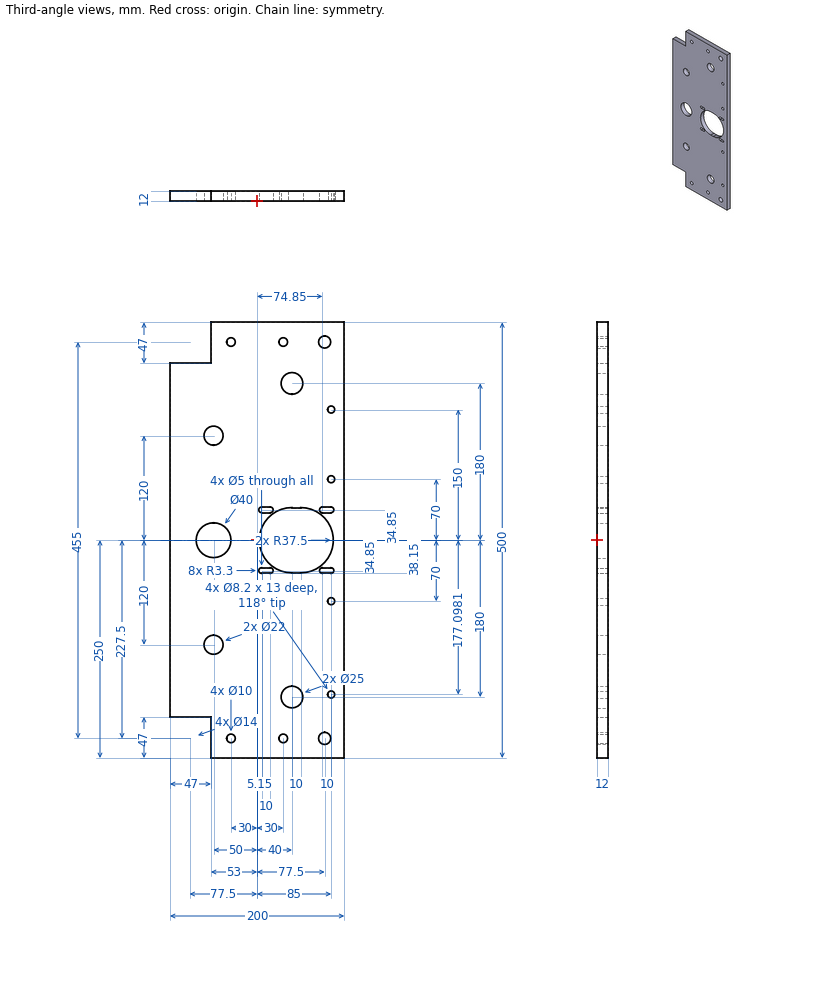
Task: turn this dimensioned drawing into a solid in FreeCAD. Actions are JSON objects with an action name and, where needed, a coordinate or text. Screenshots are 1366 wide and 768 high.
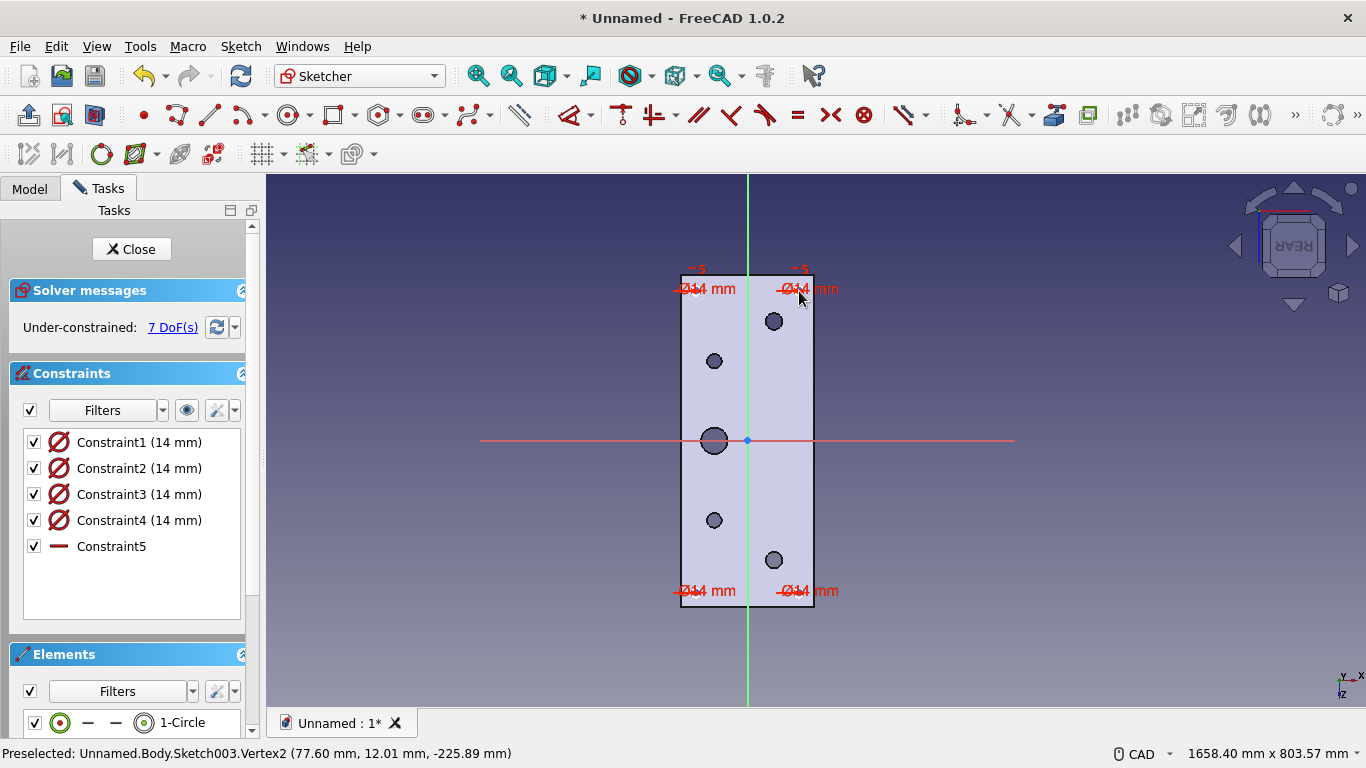
{"action": "left_click", "coordinate": [696, 291]}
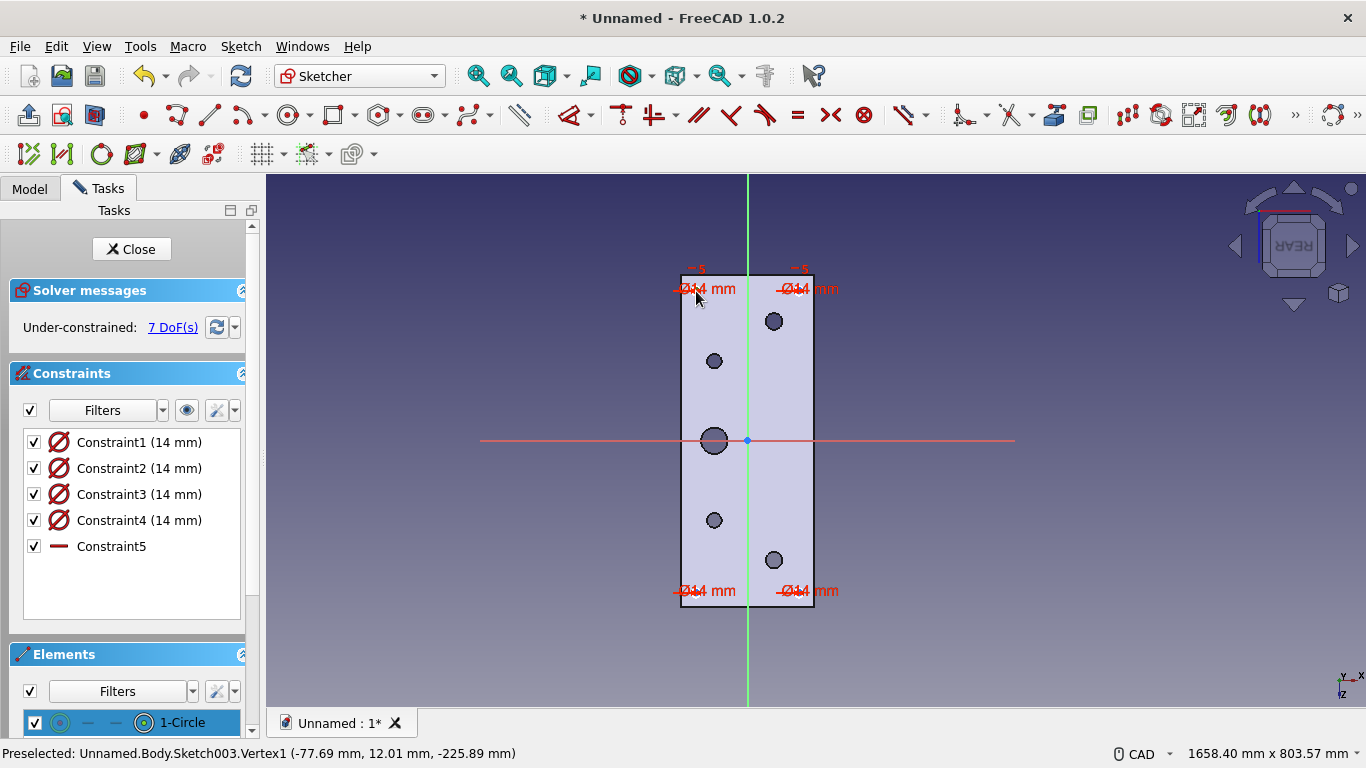
{"action": "left_click", "coordinate": [696, 593]}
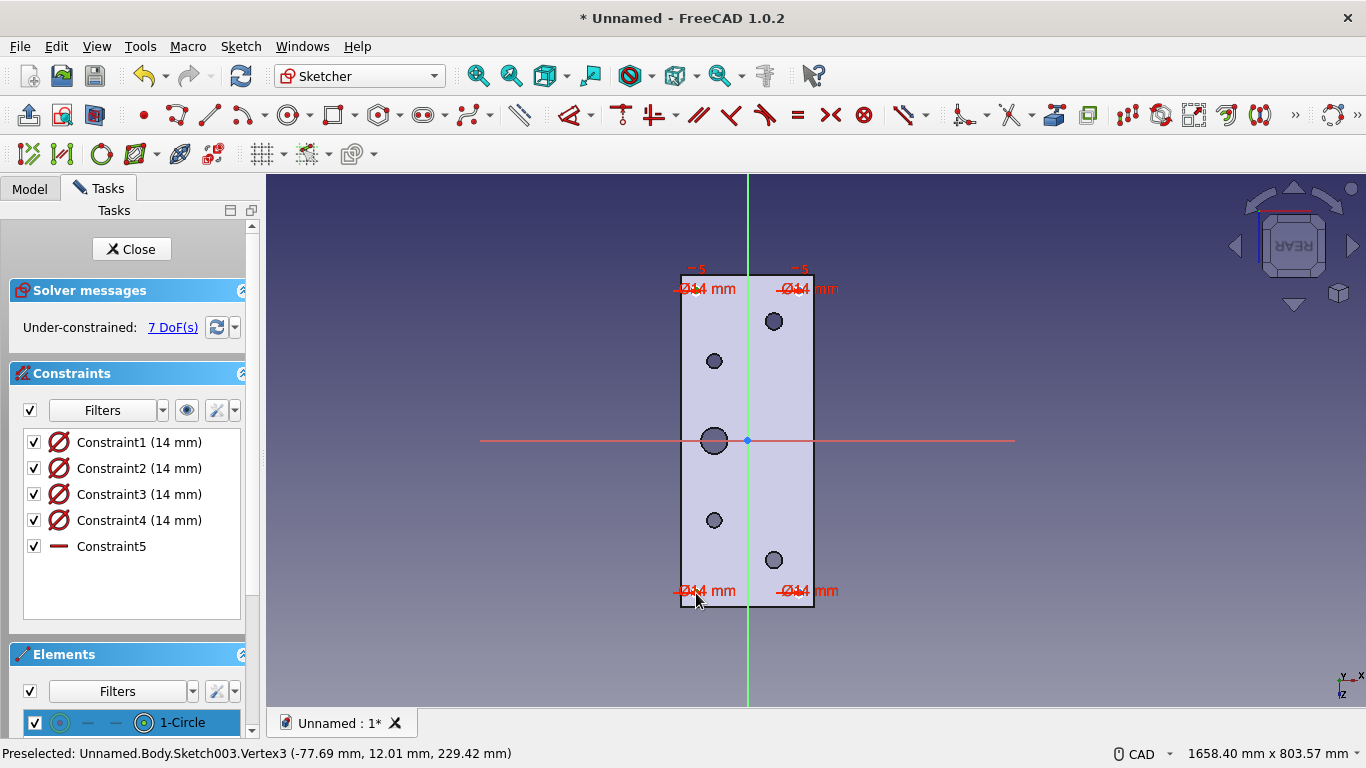
{"action": "key", "text": "v"}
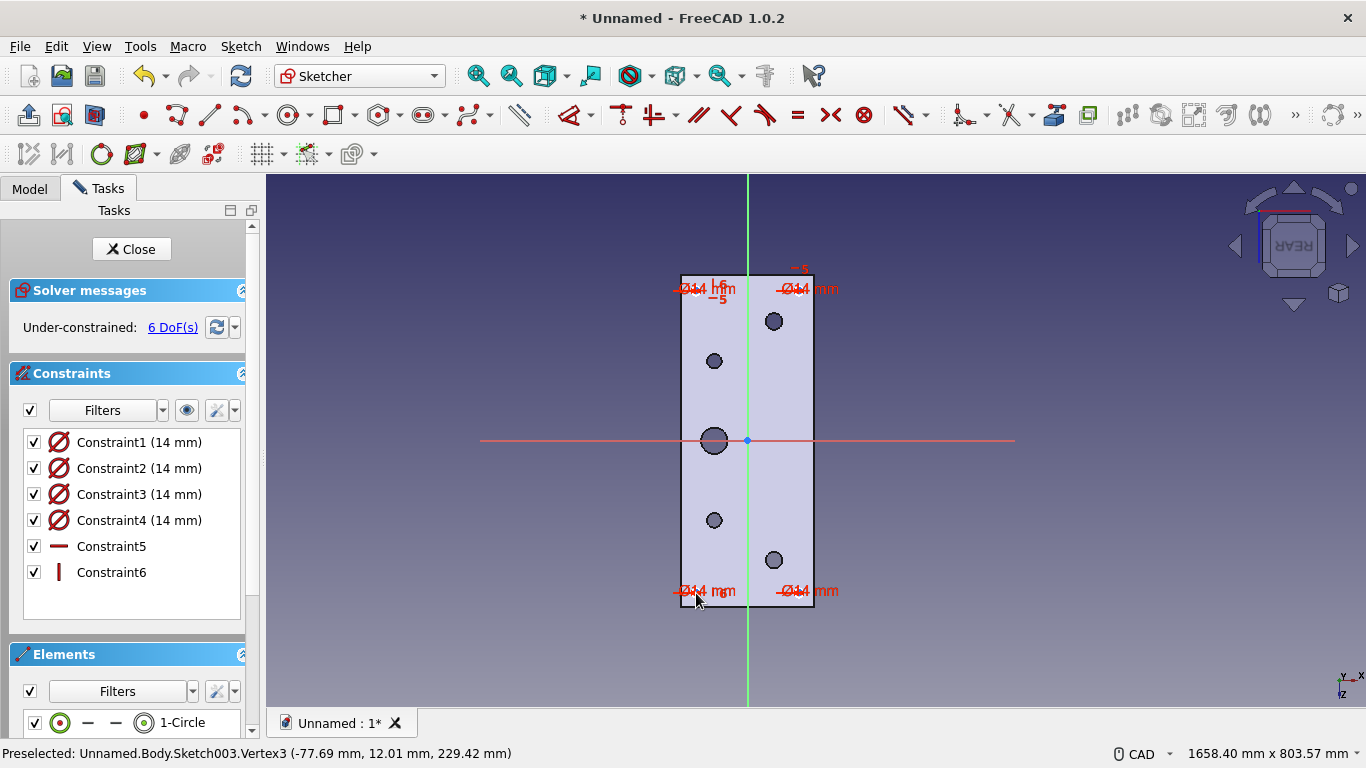
{"action": "left_click", "coordinate": [799, 291]}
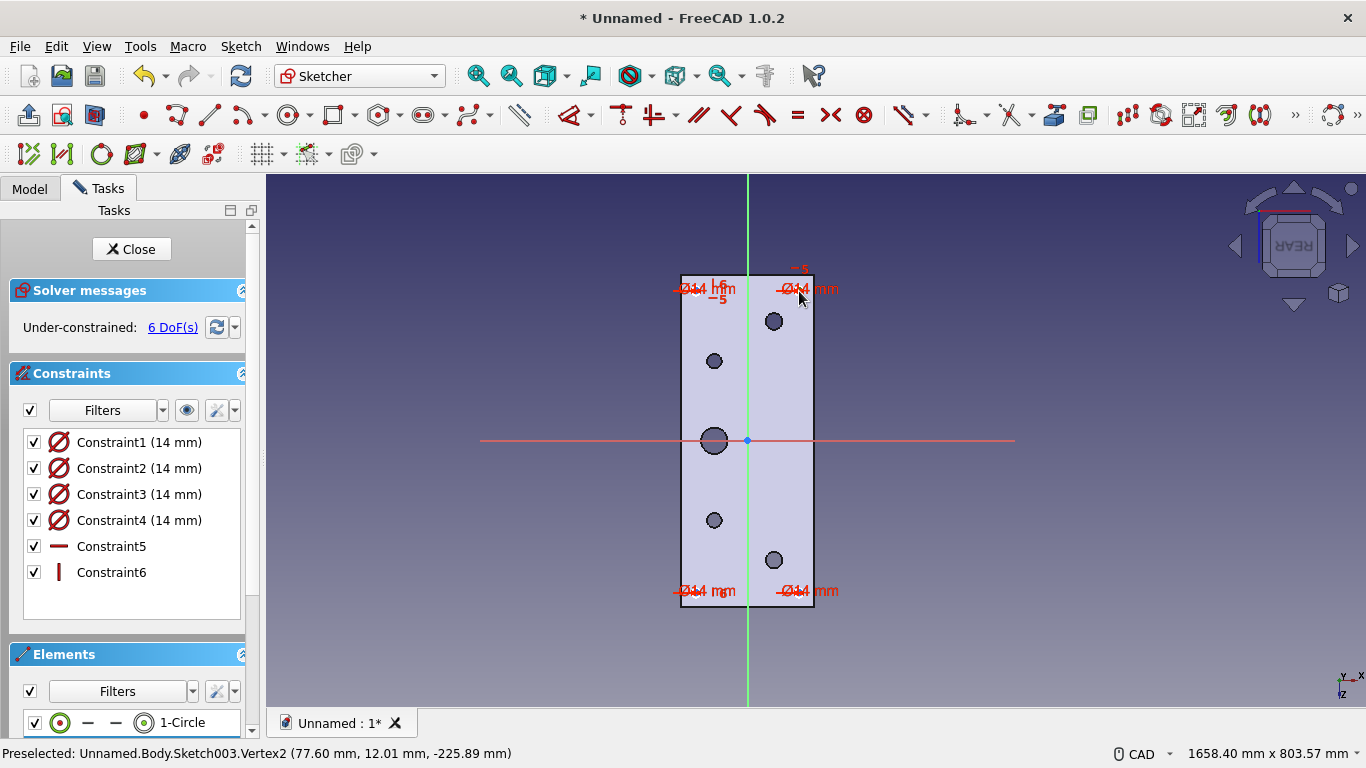
{"action": "left_click", "coordinate": [799, 593]}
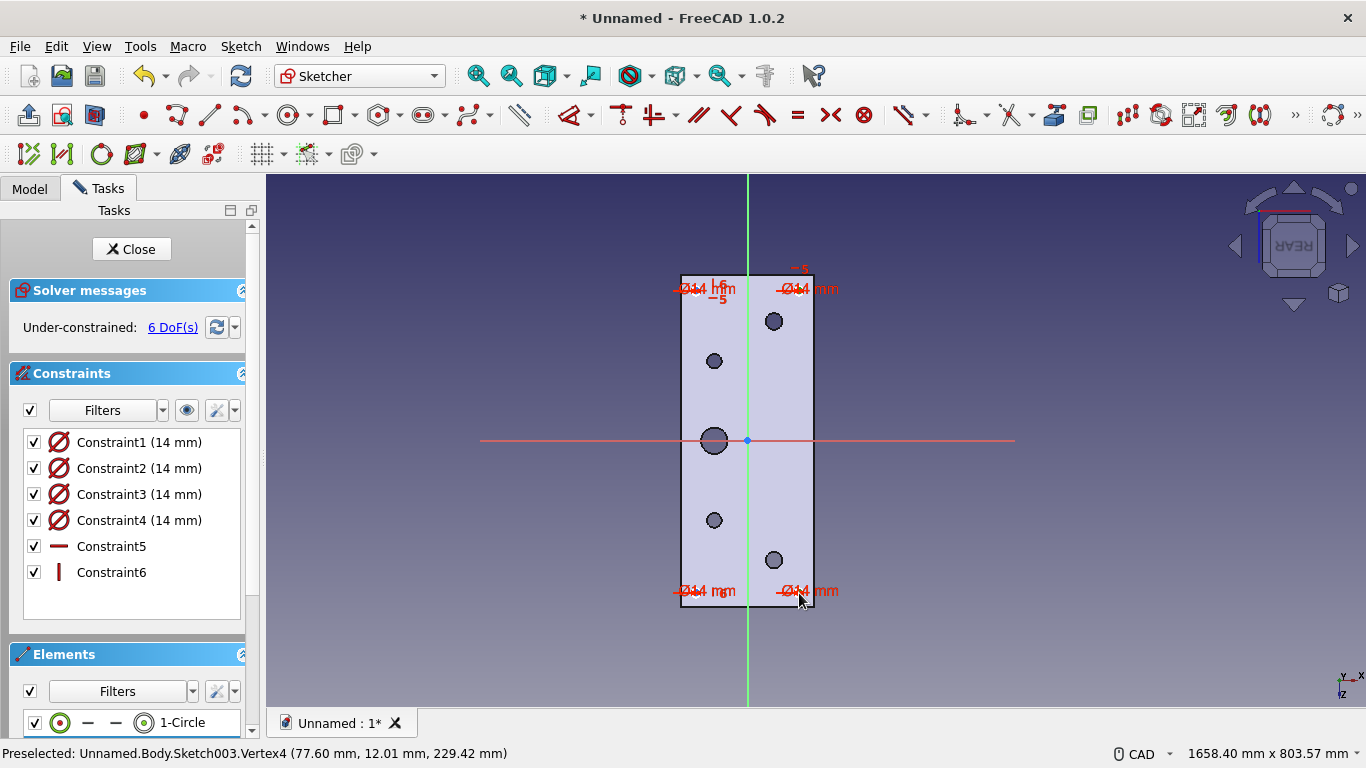
{"action": "key", "text": "v"}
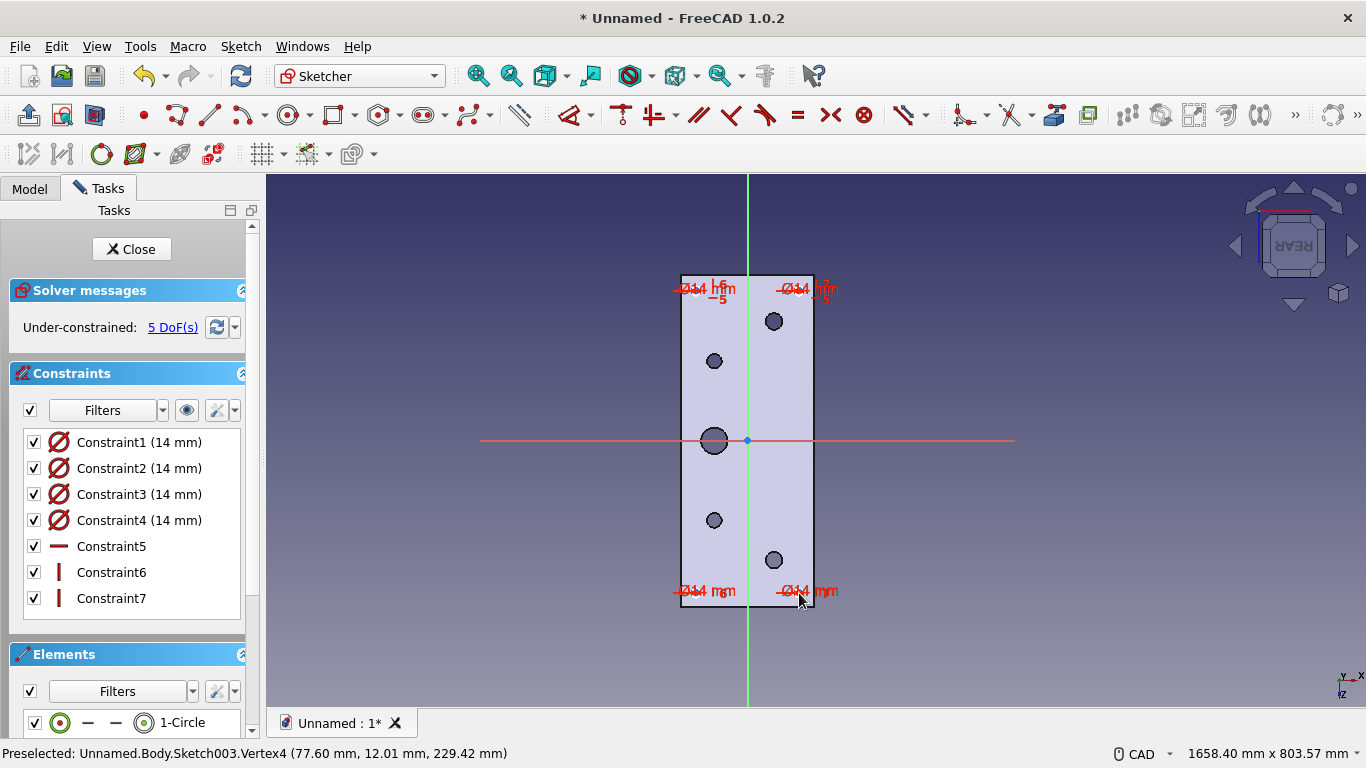
{"action": "left_click", "coordinate": [696, 593]}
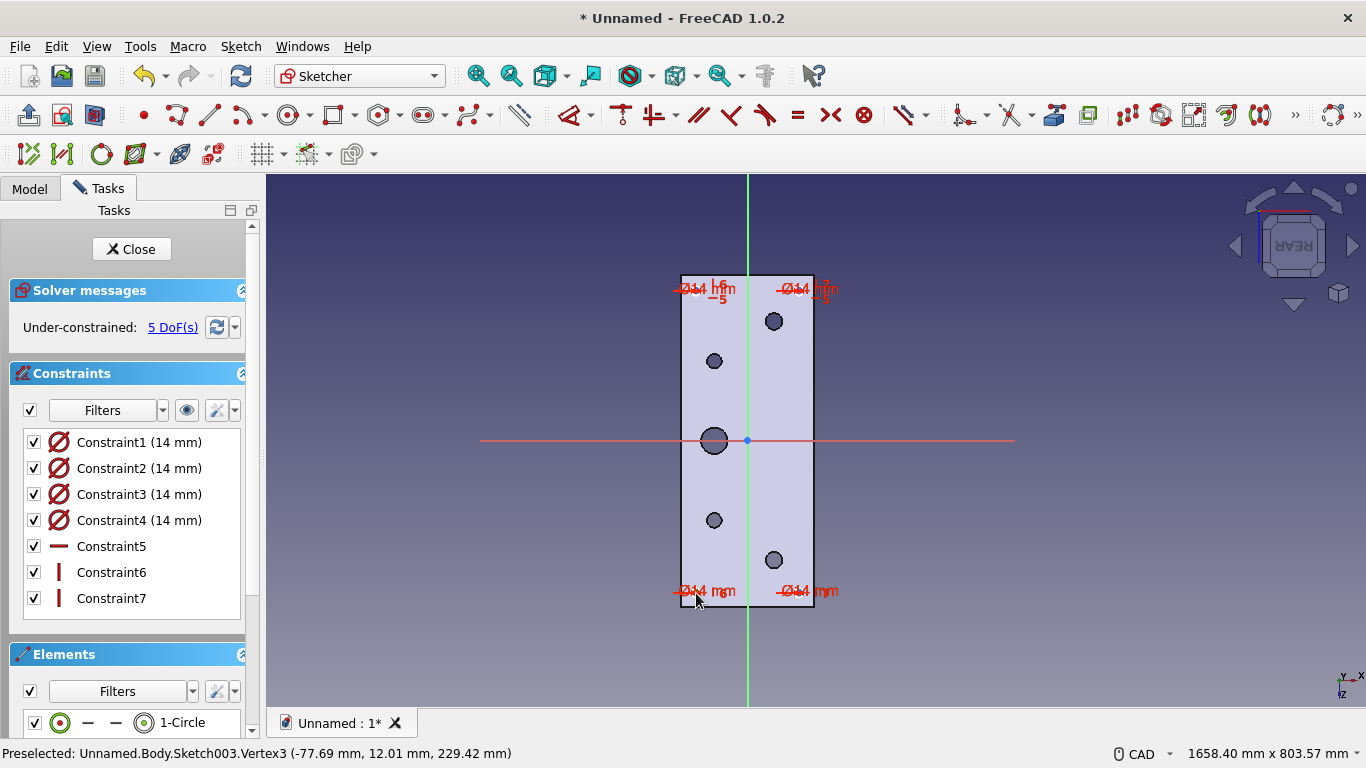
{"action": "left_click", "coordinate": [799, 593]}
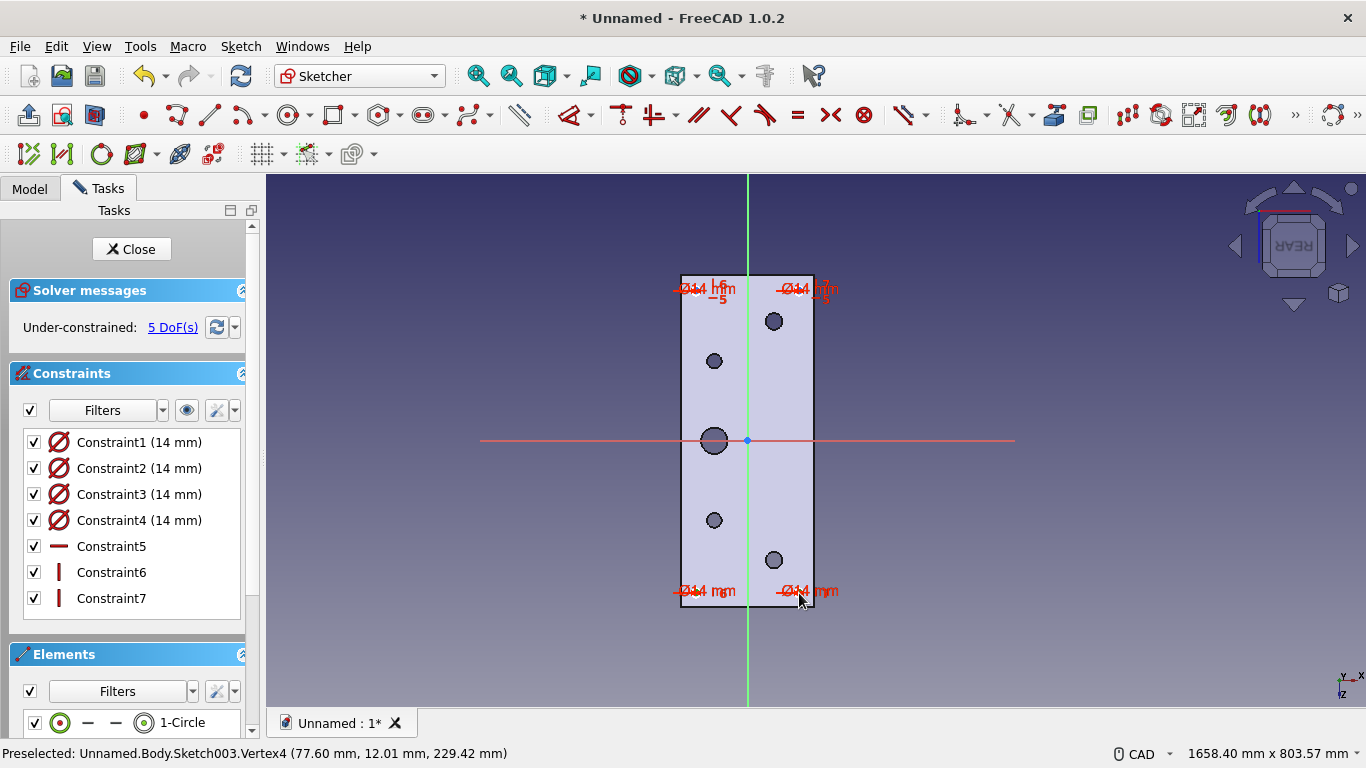
{"action": "key", "text": "h"}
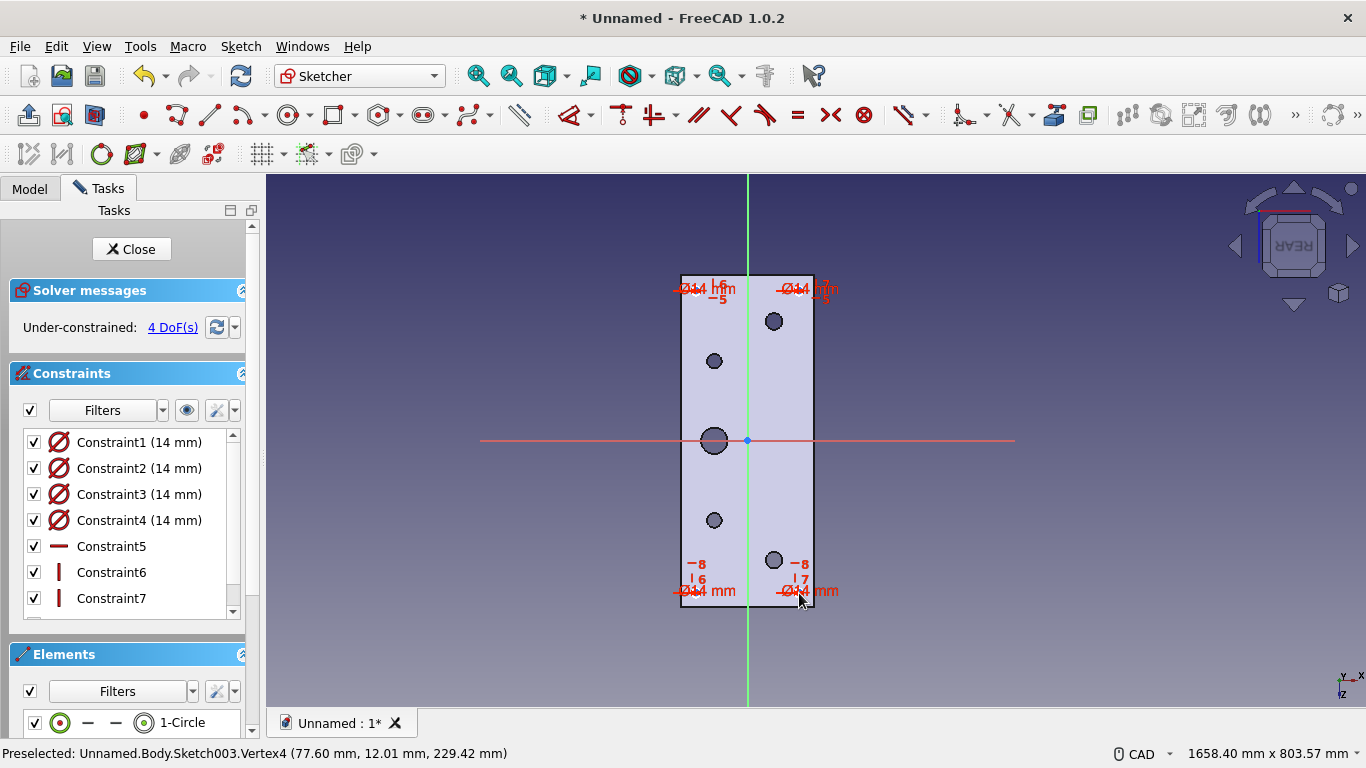
{"action": "key", "text": "d"}